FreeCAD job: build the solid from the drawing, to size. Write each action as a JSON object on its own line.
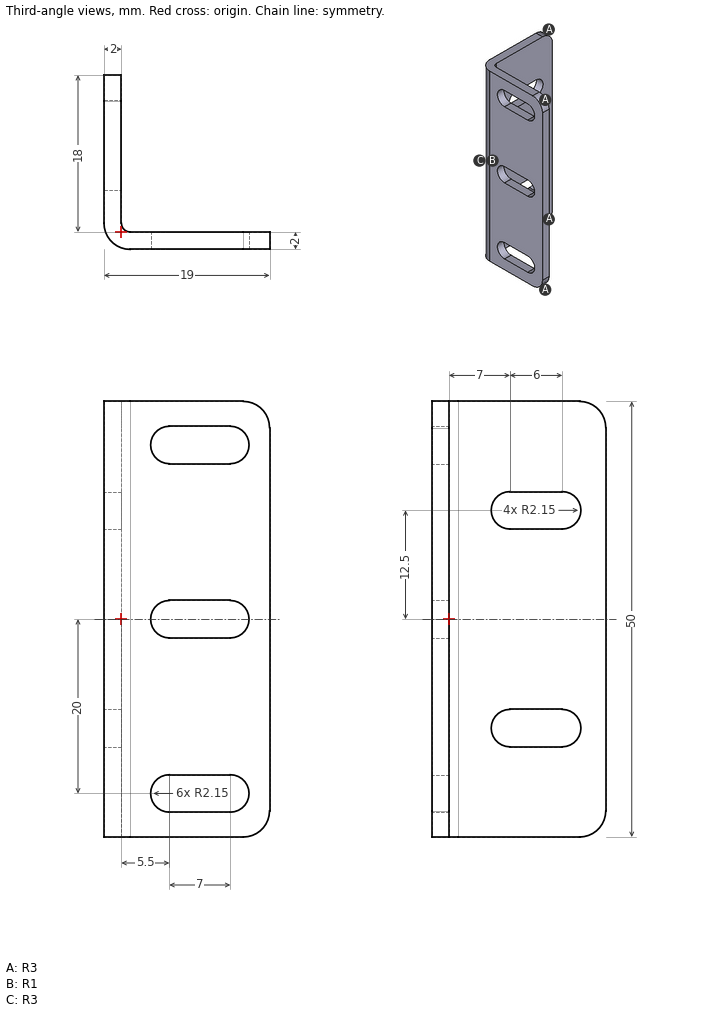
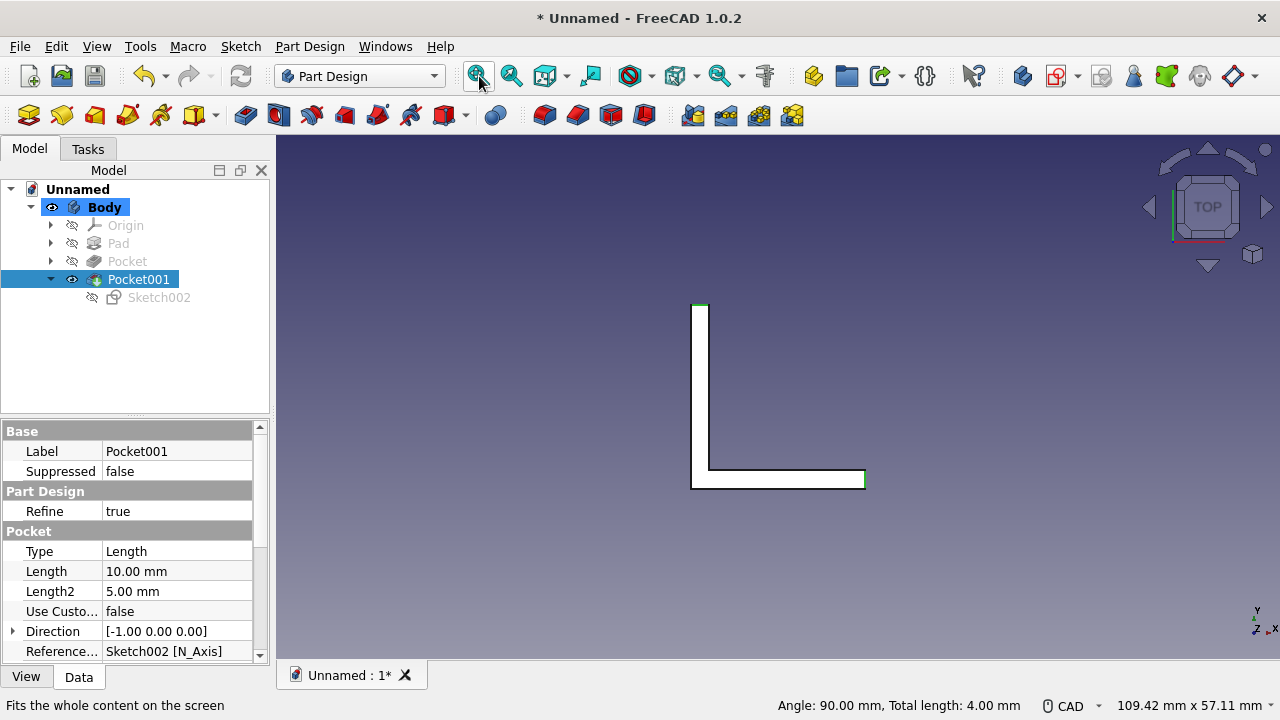
{"action": "key", "text": "1"}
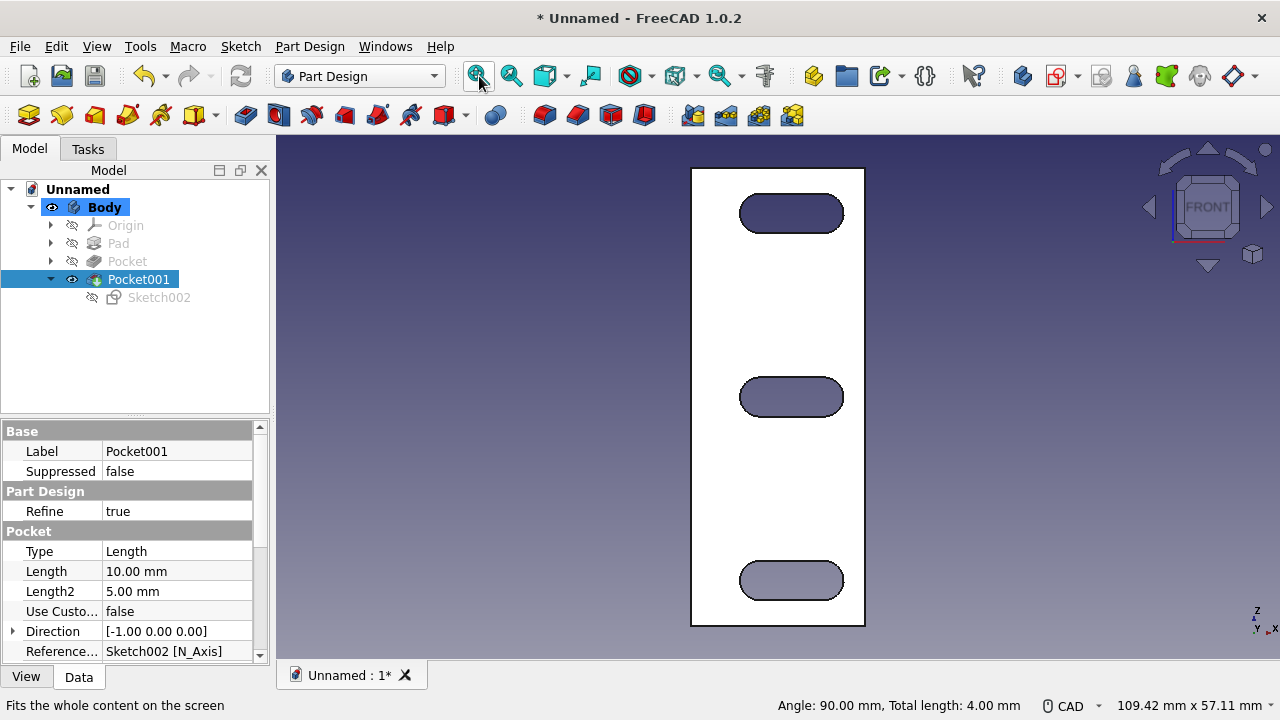
{"action": "scroll", "coordinate": [700, 625], "scroll_direction": "up", "scroll_amount": 4}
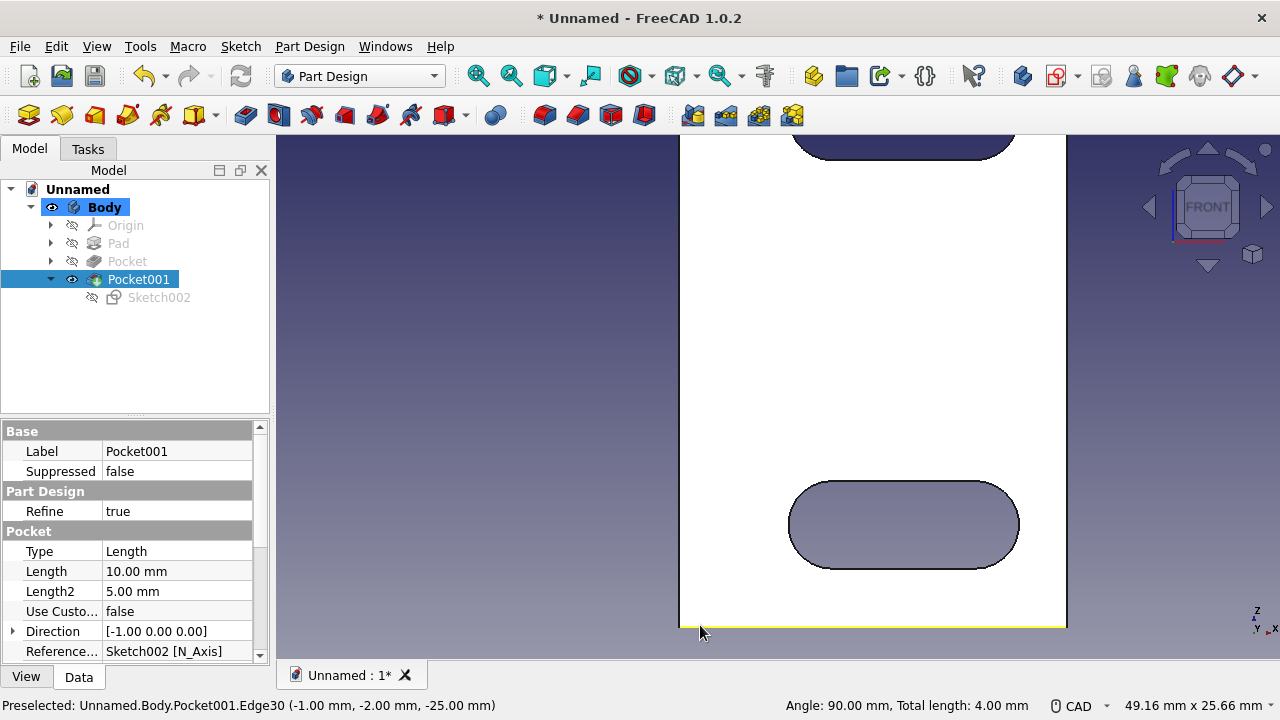
{"action": "left_click", "coordinate": [479, 76]}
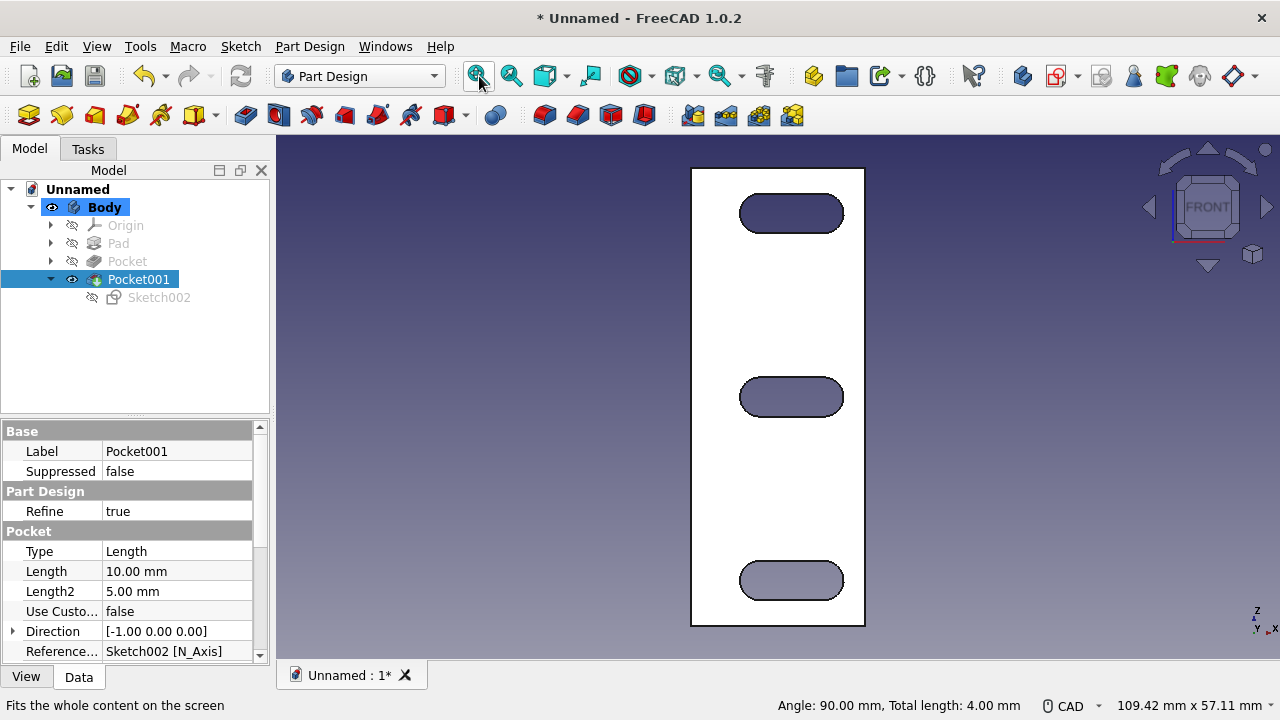
{"action": "key", "text": "3"}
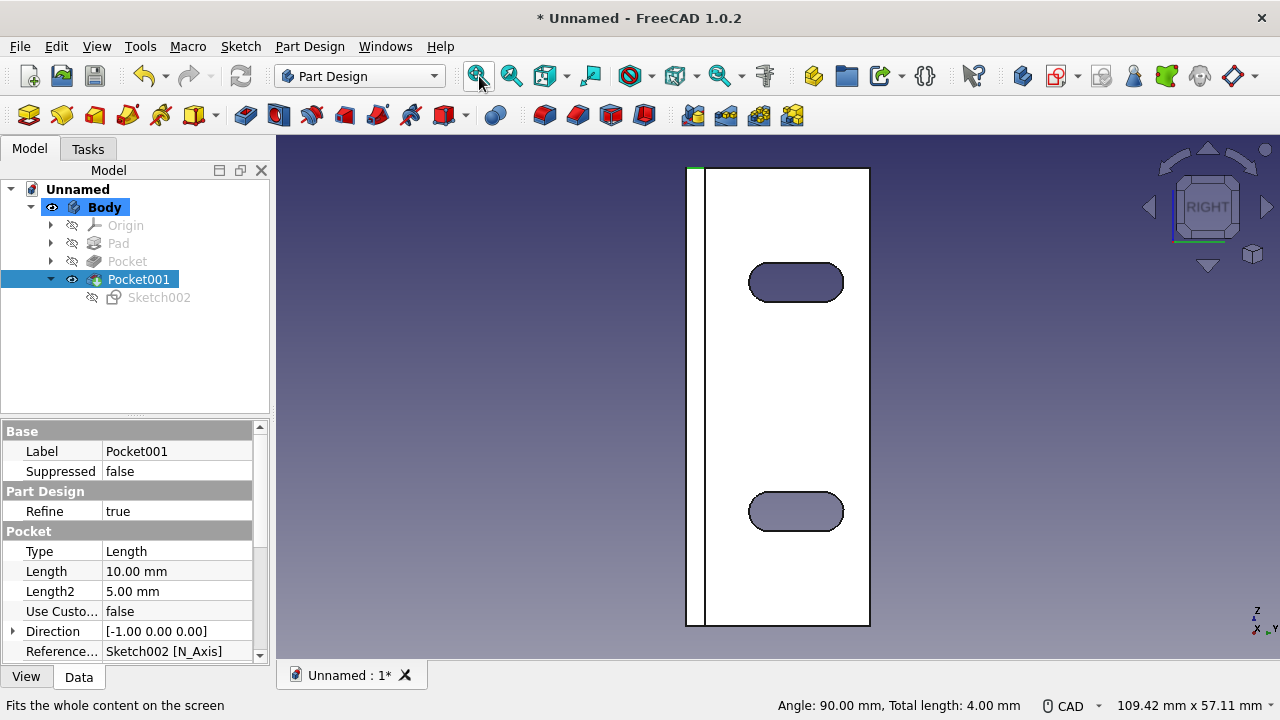
{"action": "left_click", "coordinate": [695, 625], "text": "ctrl"}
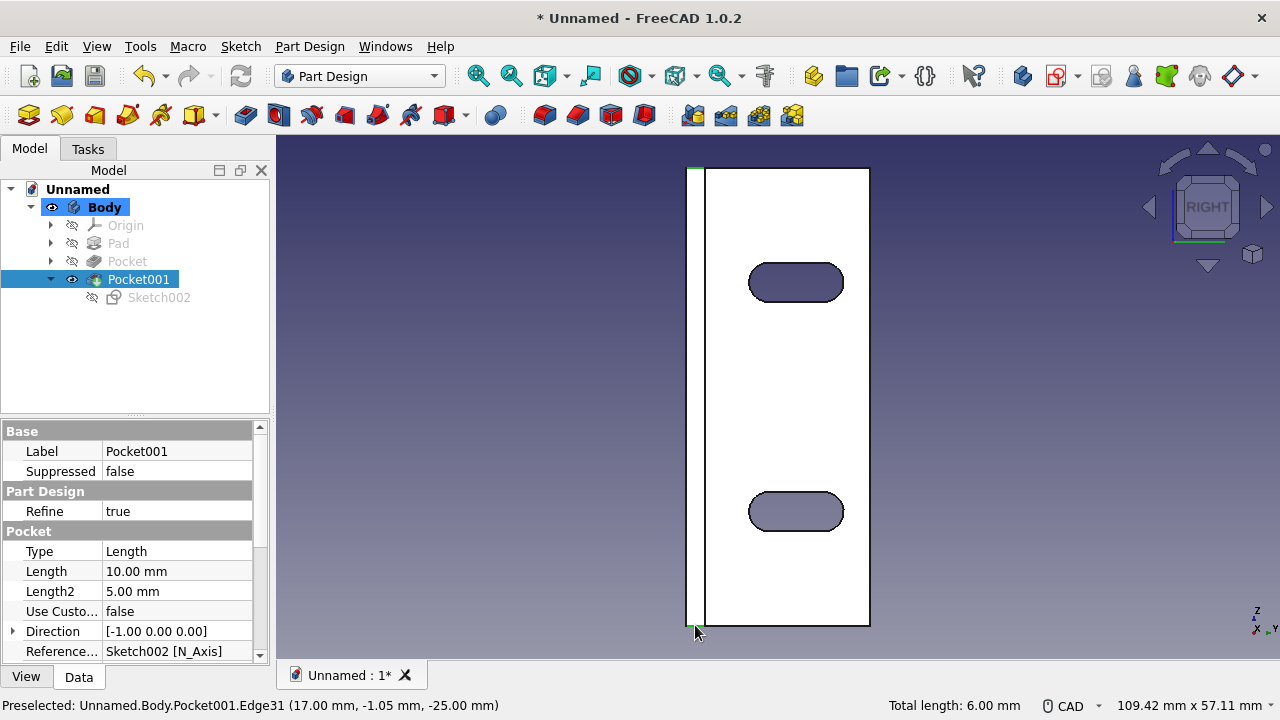
{"action": "scroll", "coordinate": [870, 625], "scroll_direction": "up", "scroll_amount": 4}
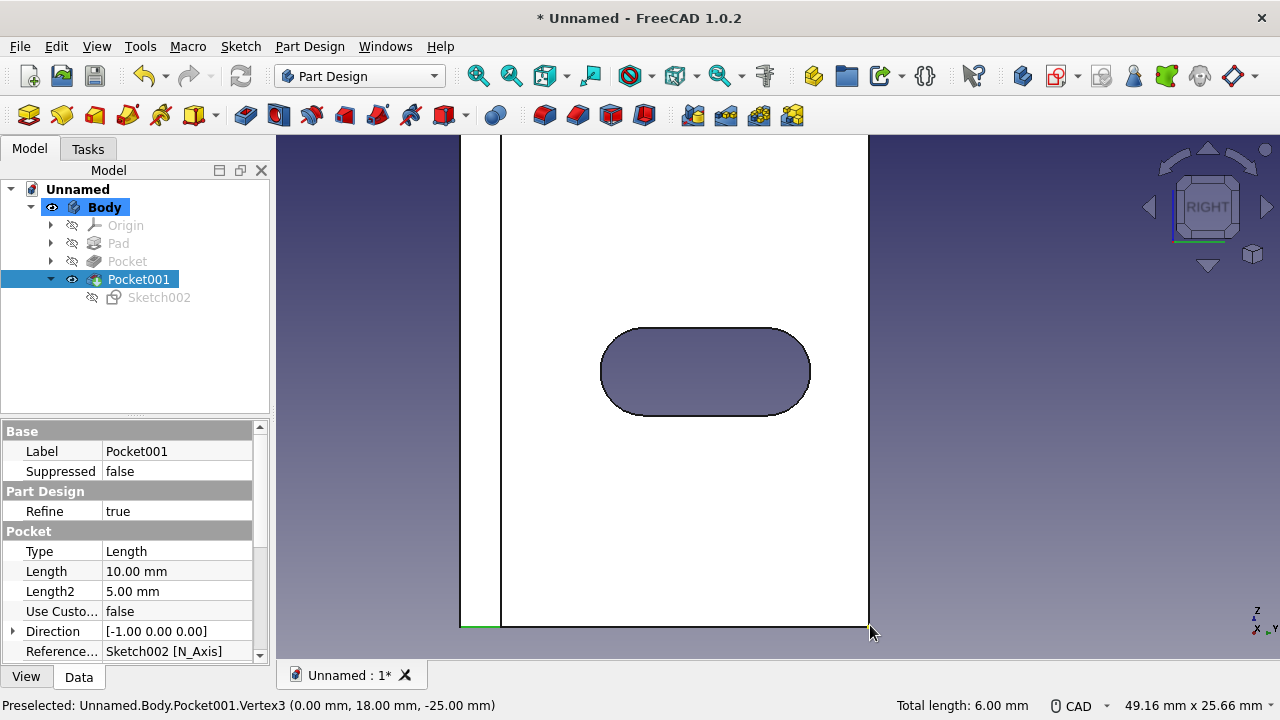
{"action": "left_click", "coordinate": [479, 76]}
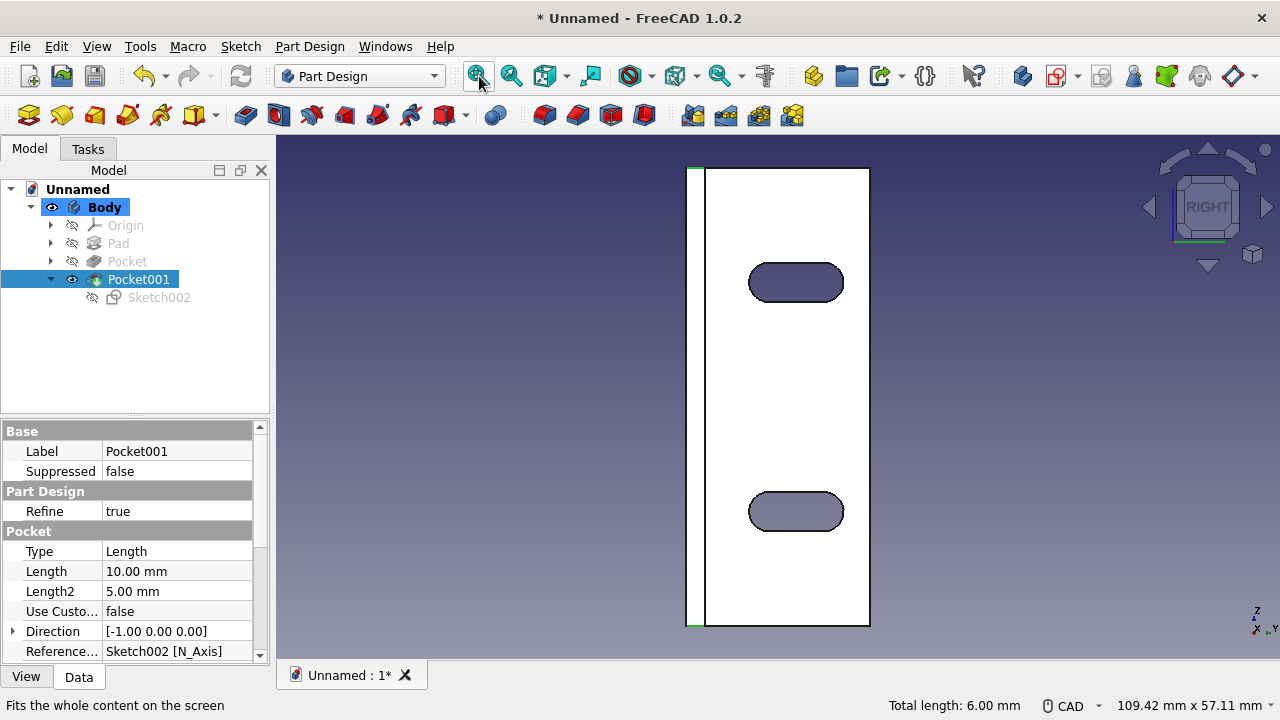
{"action": "key", "text": "5"}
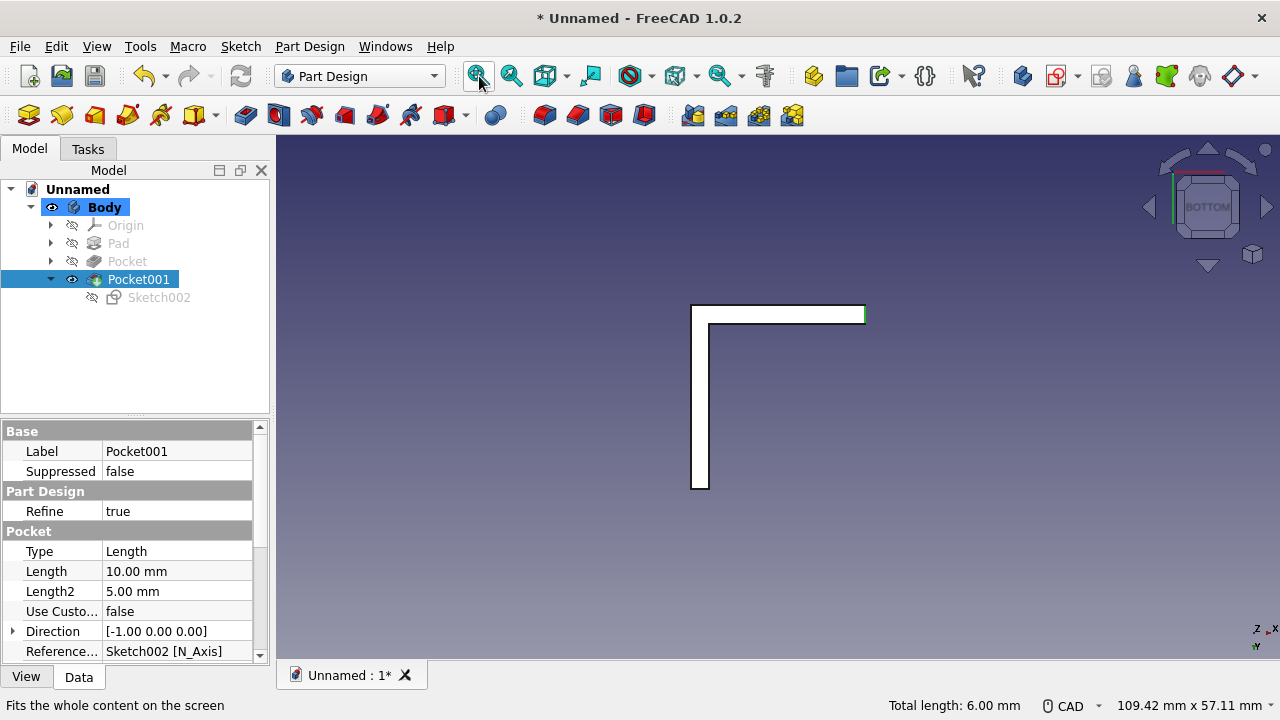
{"action": "left_click", "coordinate": [479, 76]}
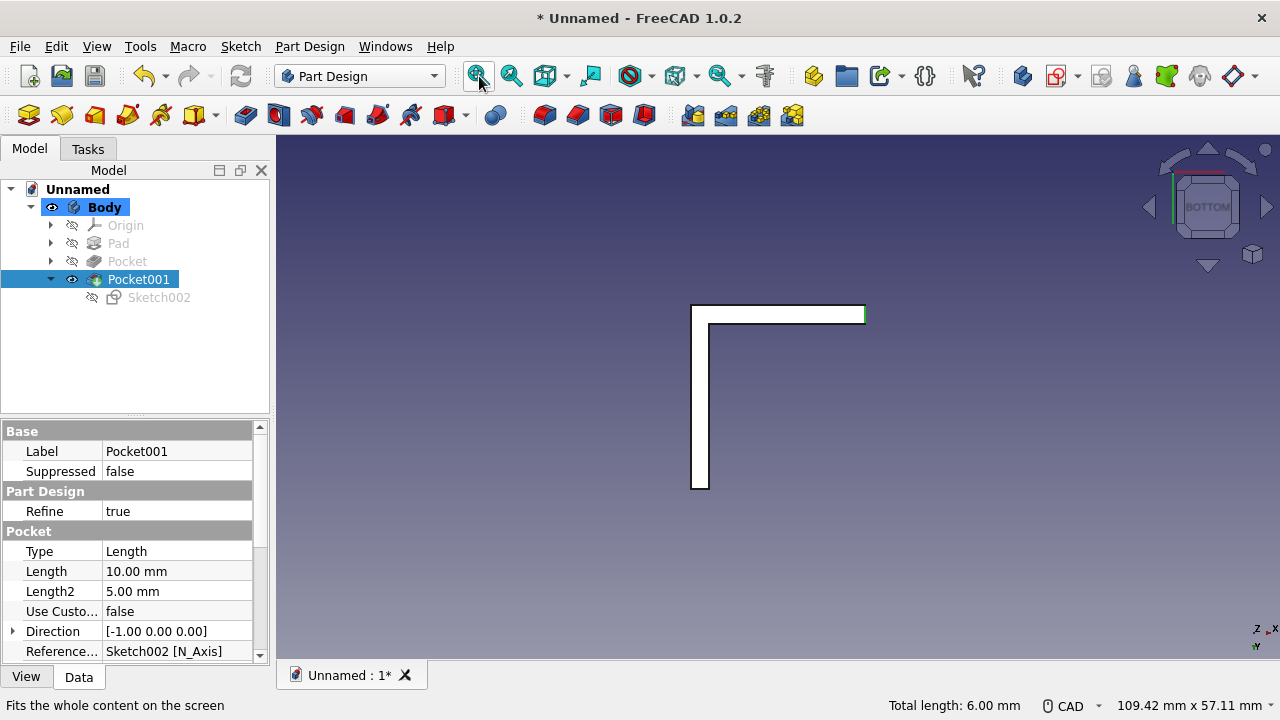
{"action": "left_click", "coordinate": [700, 488], "text": "ctrl"}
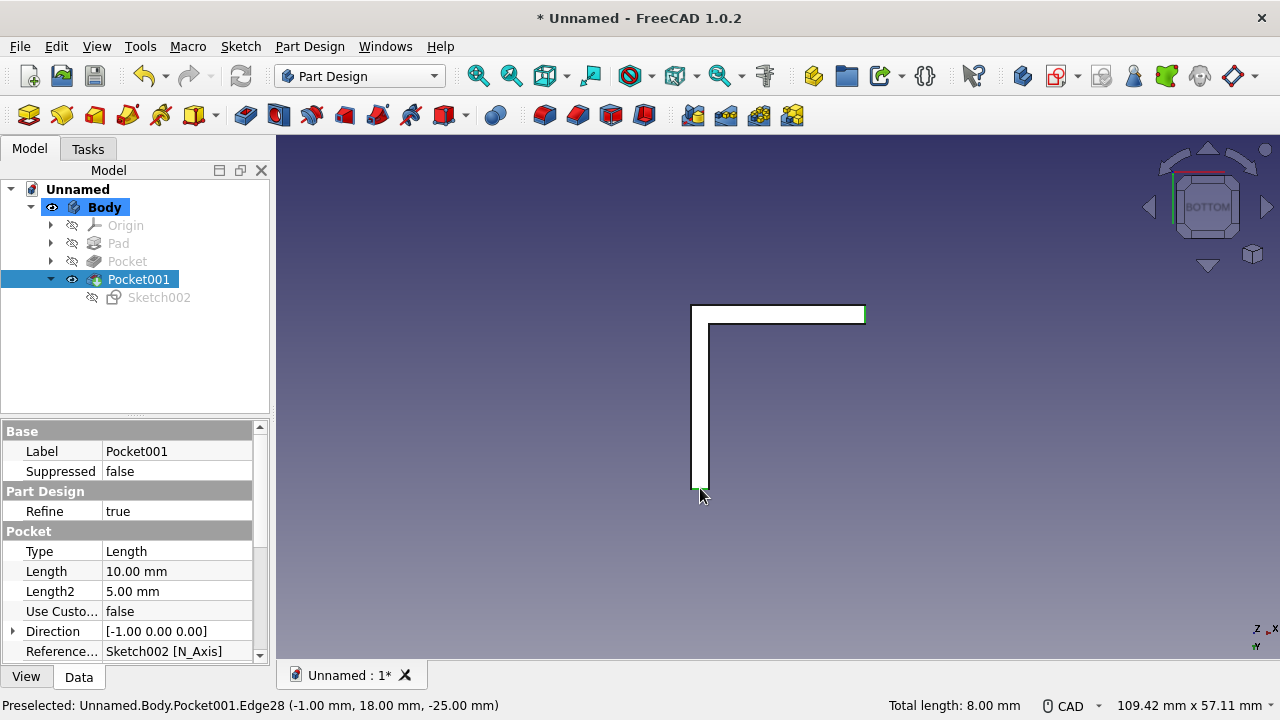
{"action": "left_click", "coordinate": [545, 116]}